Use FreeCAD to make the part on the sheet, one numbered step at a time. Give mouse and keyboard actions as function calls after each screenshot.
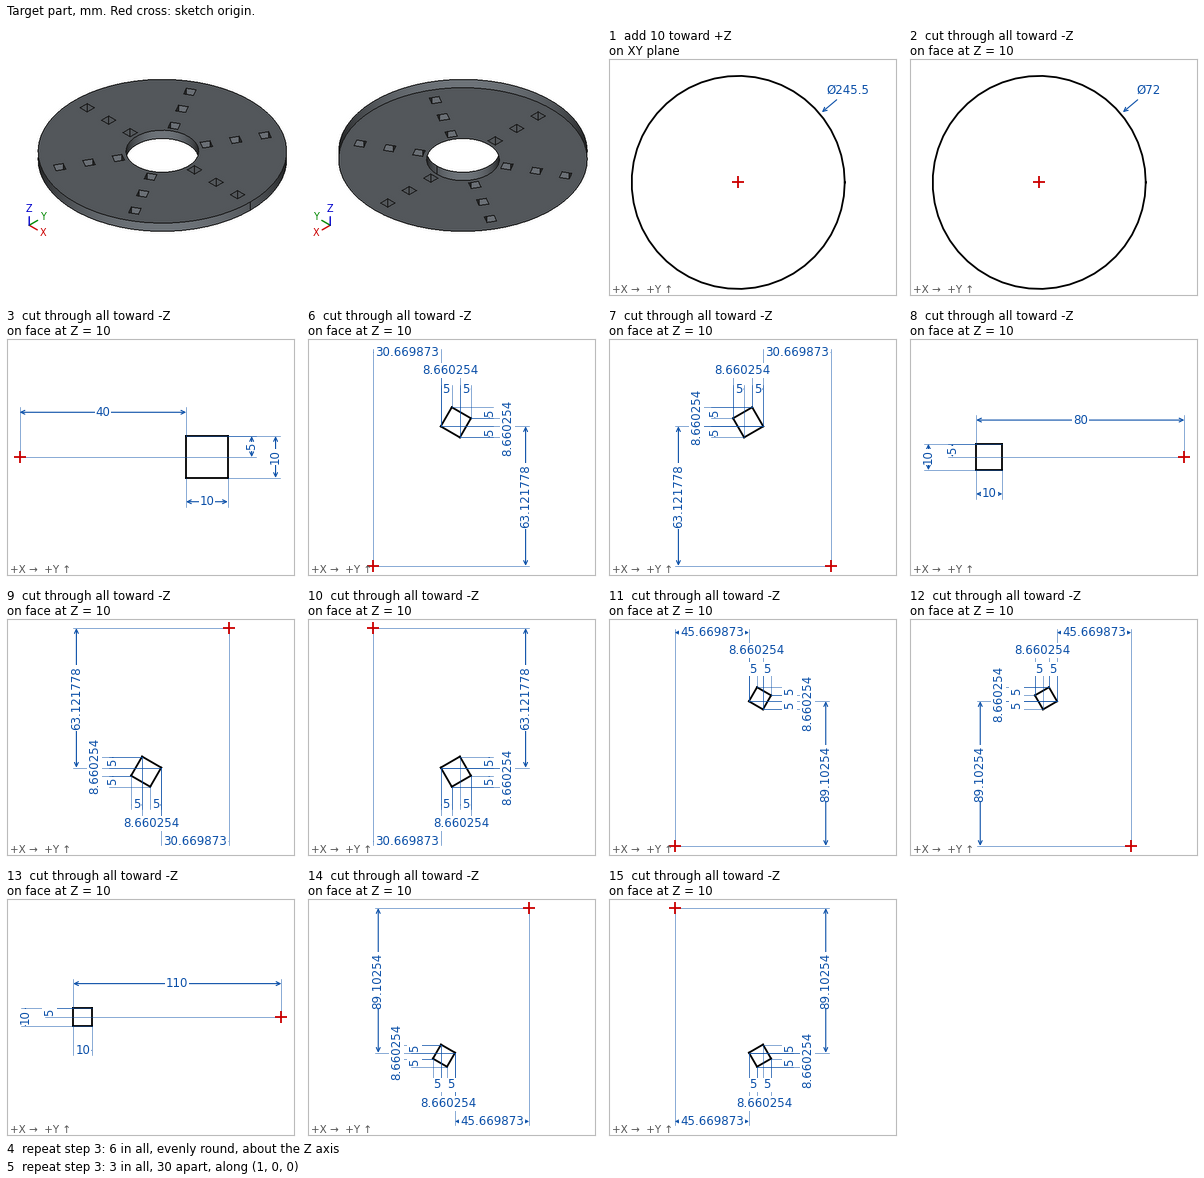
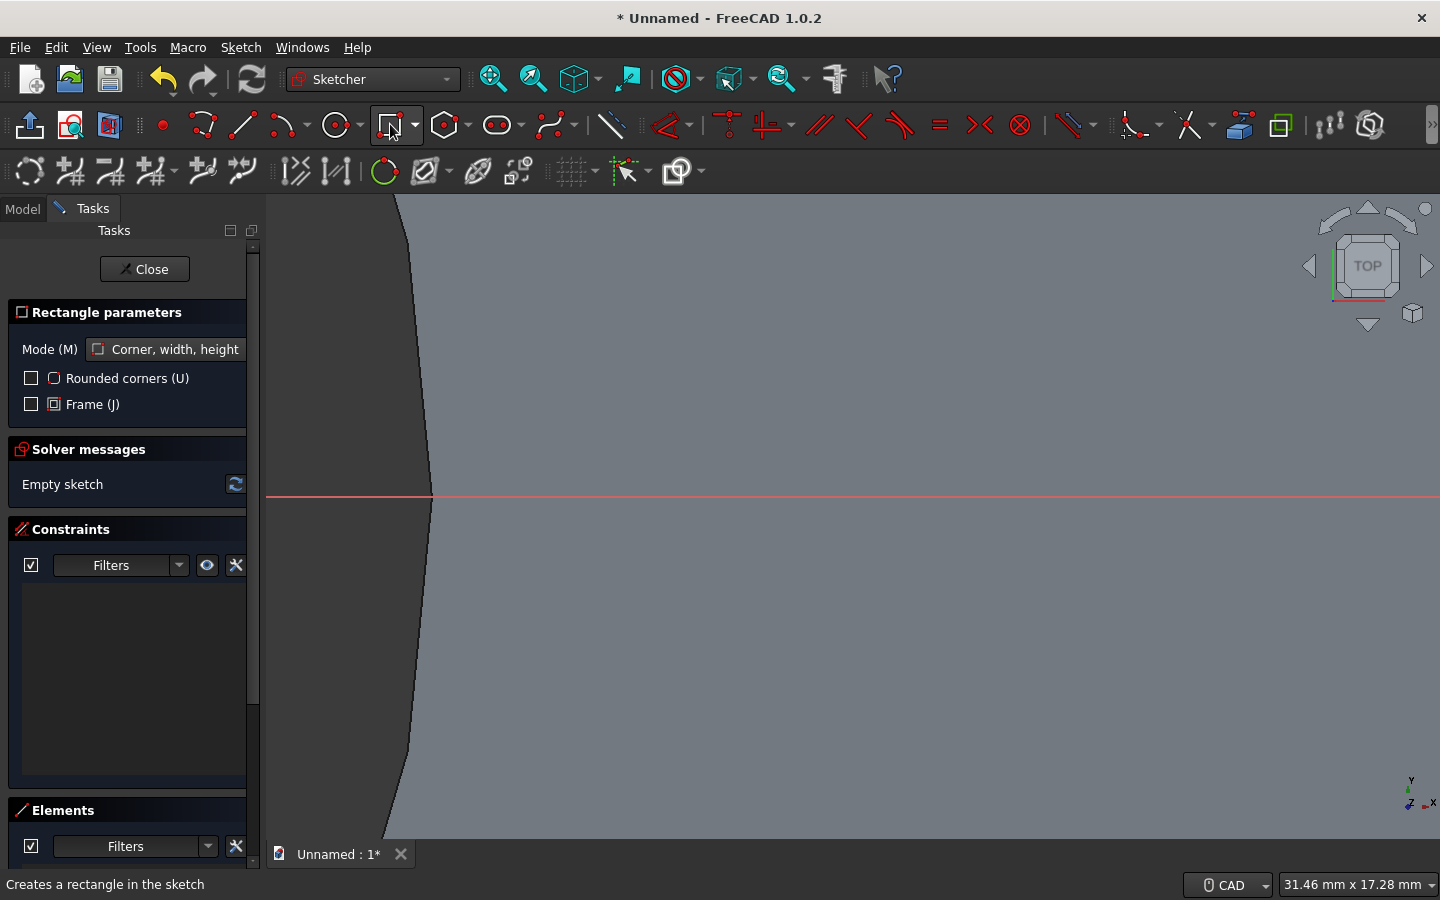
click(581, 311)
move(954, 684)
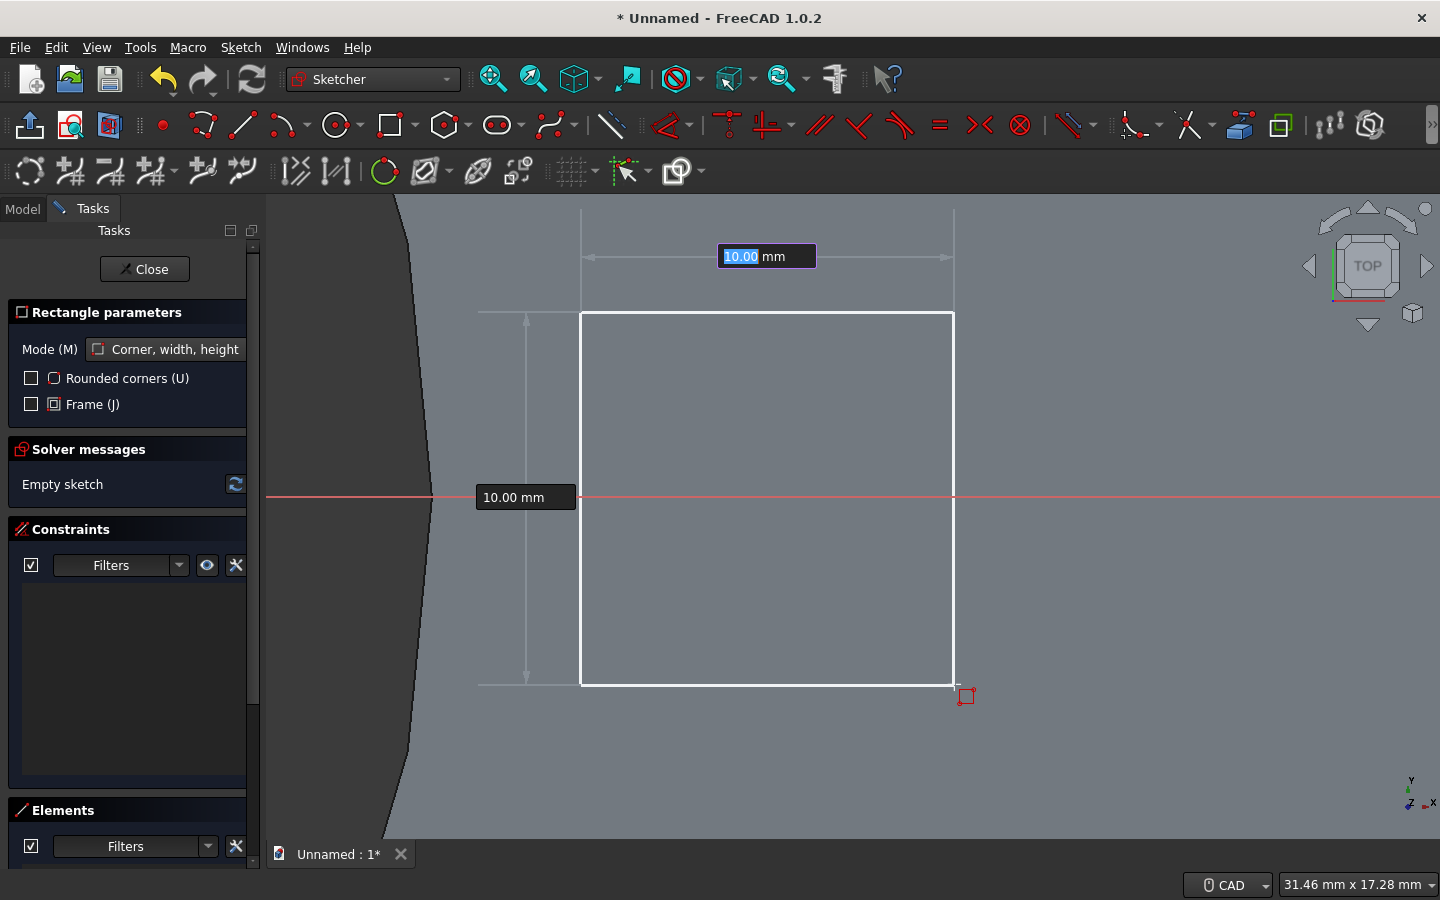
text(10)
key(Tab)
text(10)
key(Return)
key(Escape)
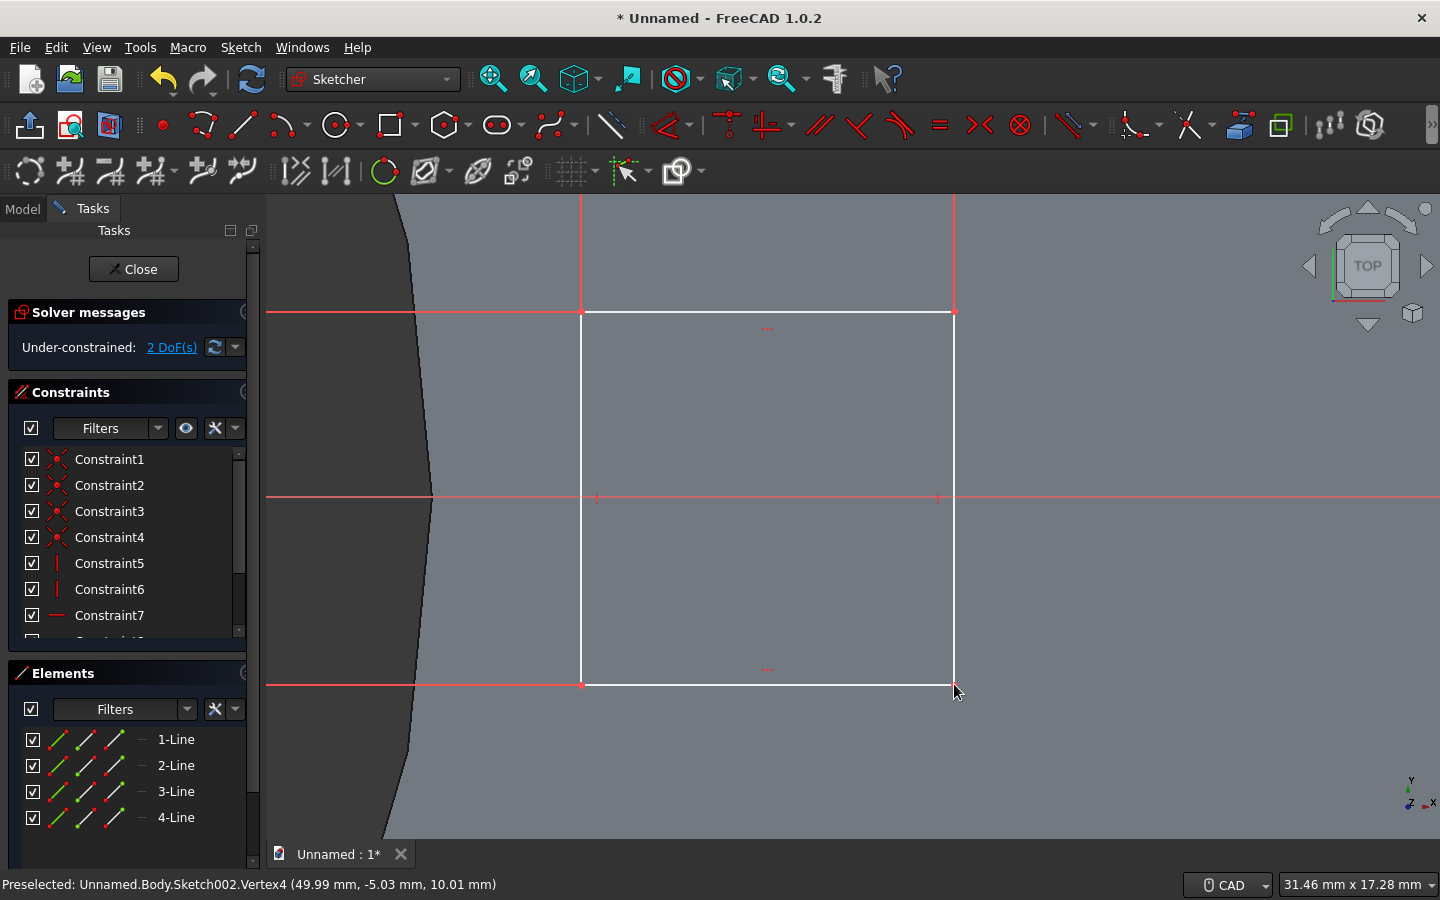
key(d)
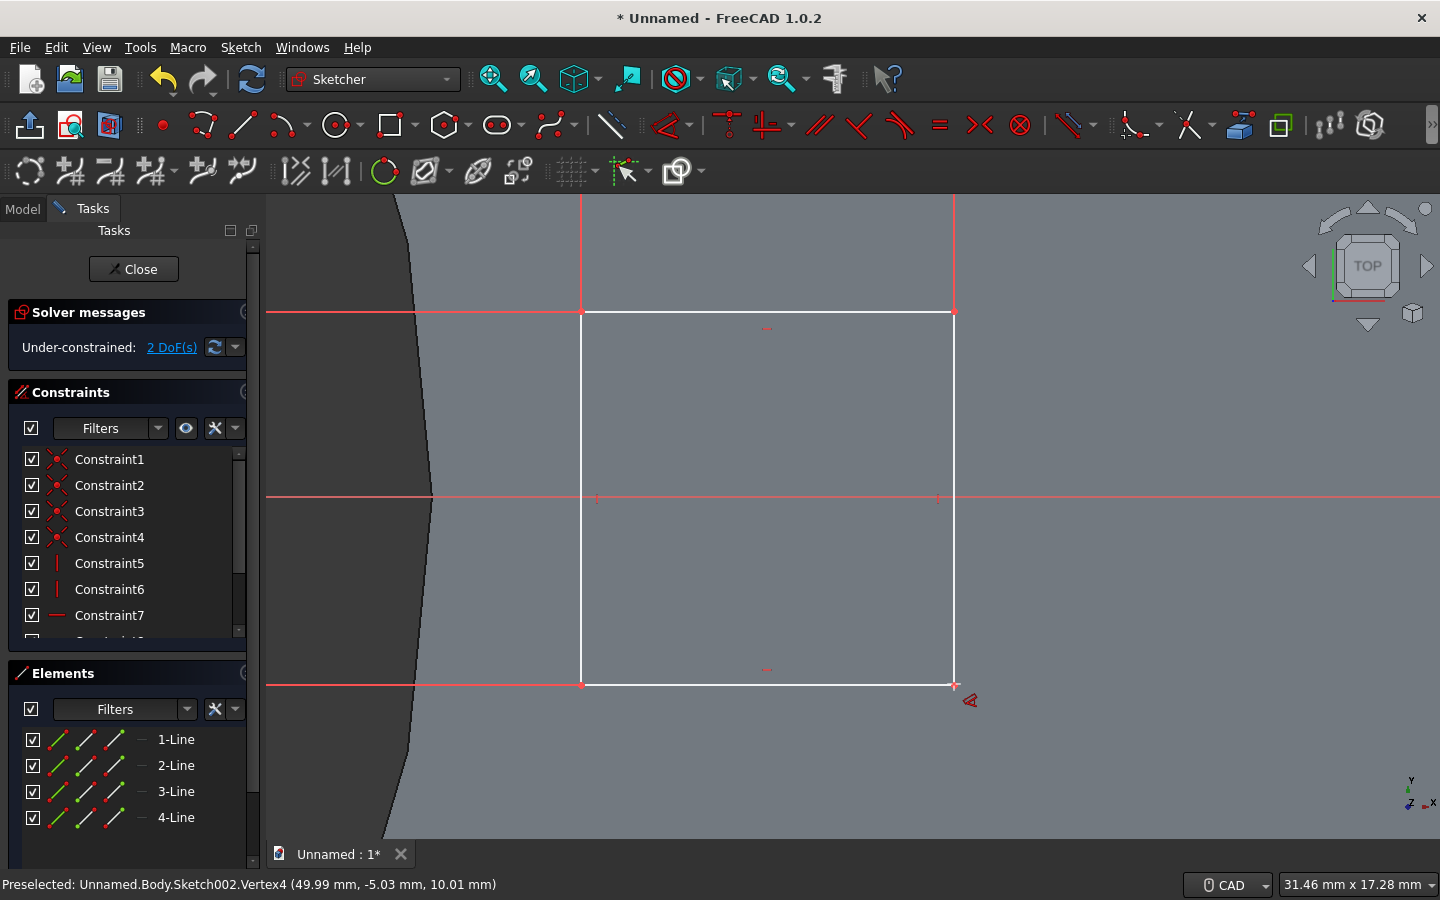
click(581, 312)
click(615, 405)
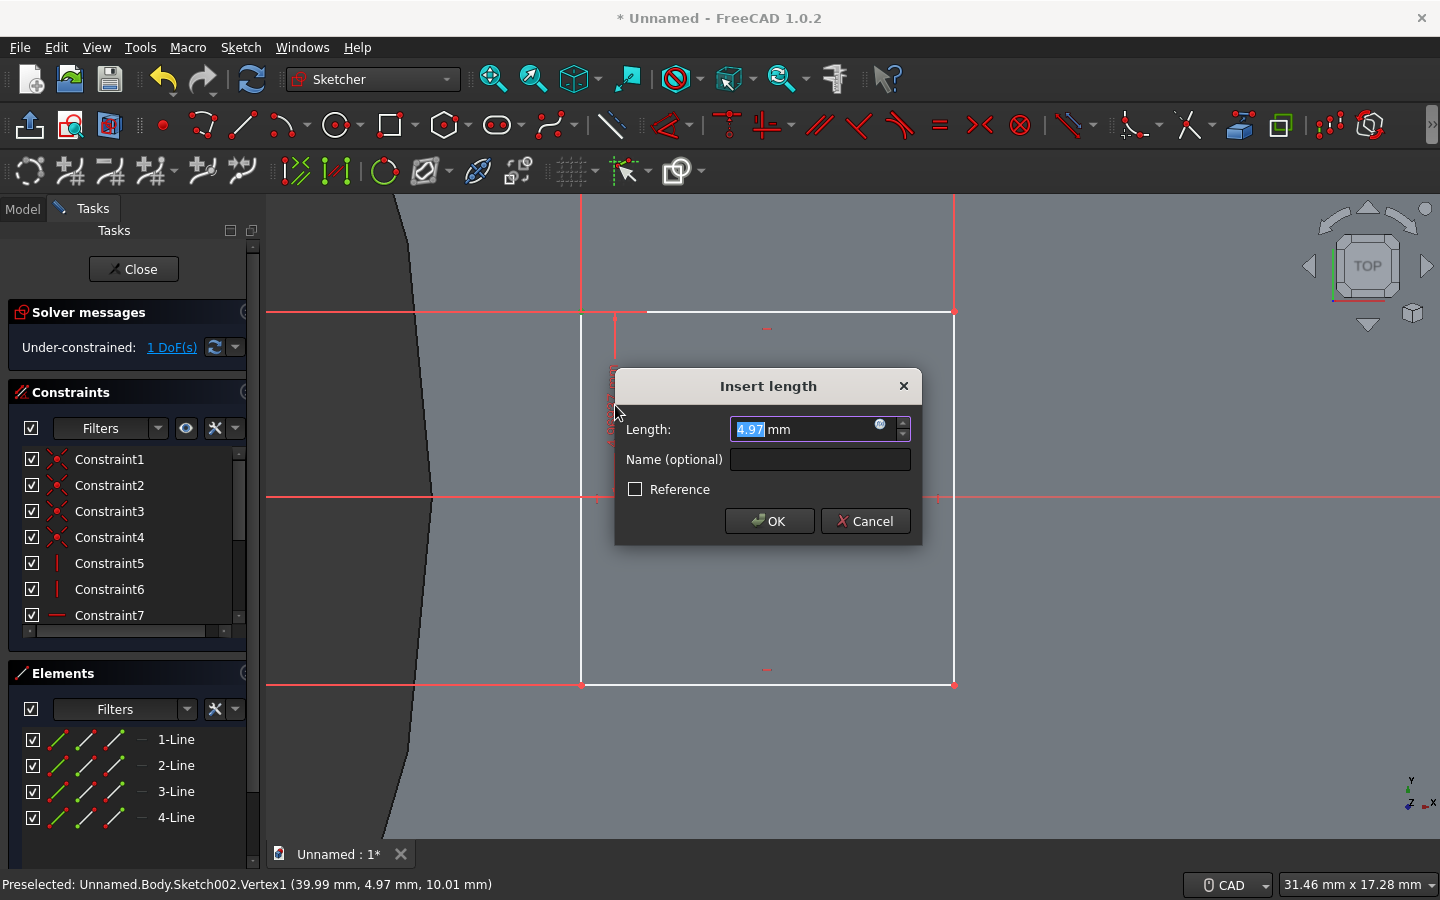
text(5)
key(Return)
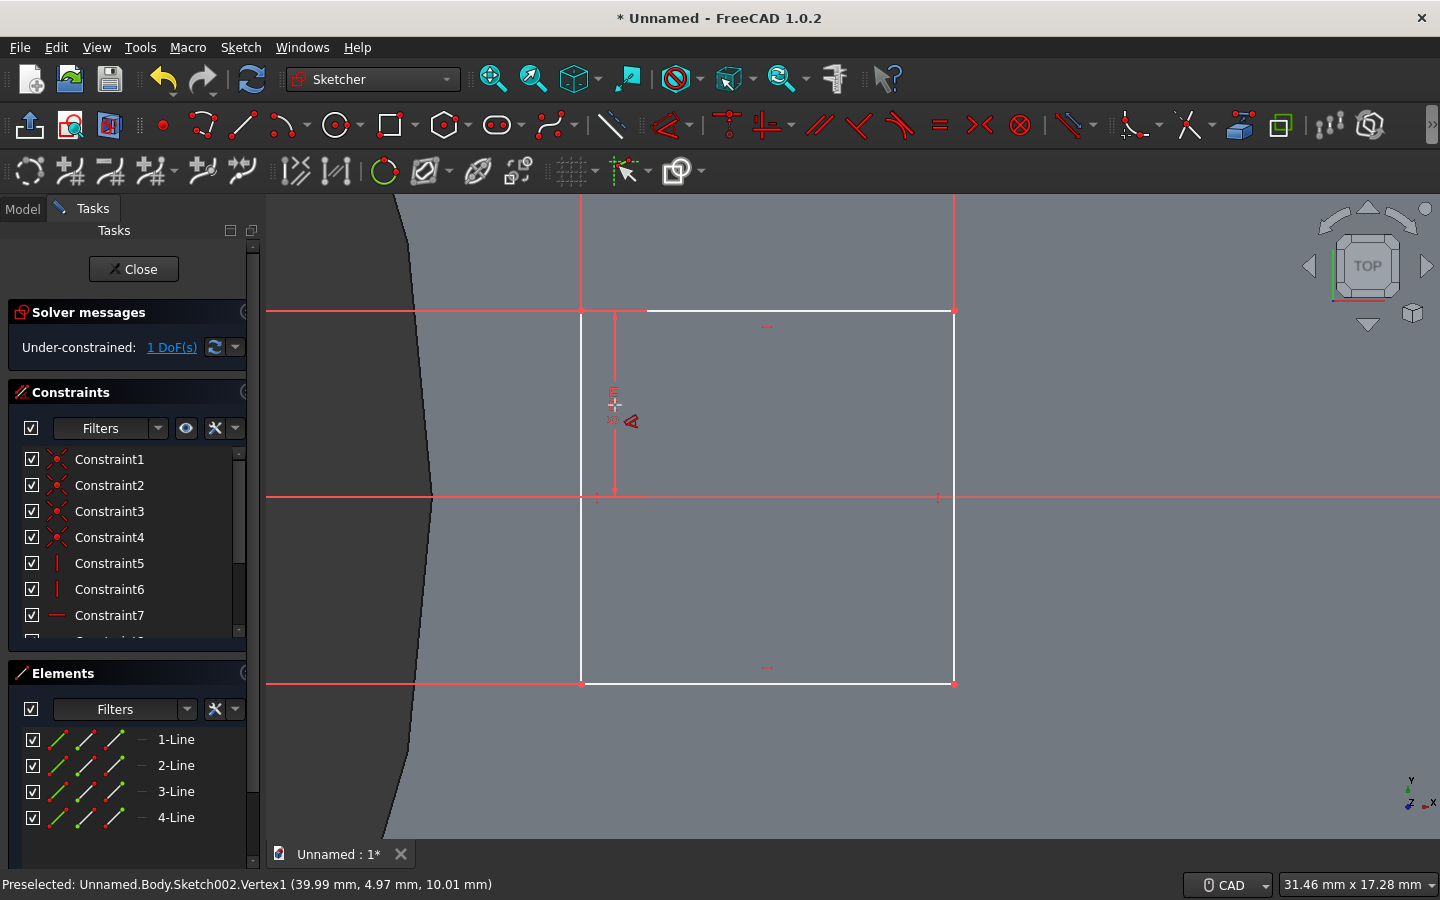
click(581, 311)
click(437, 277)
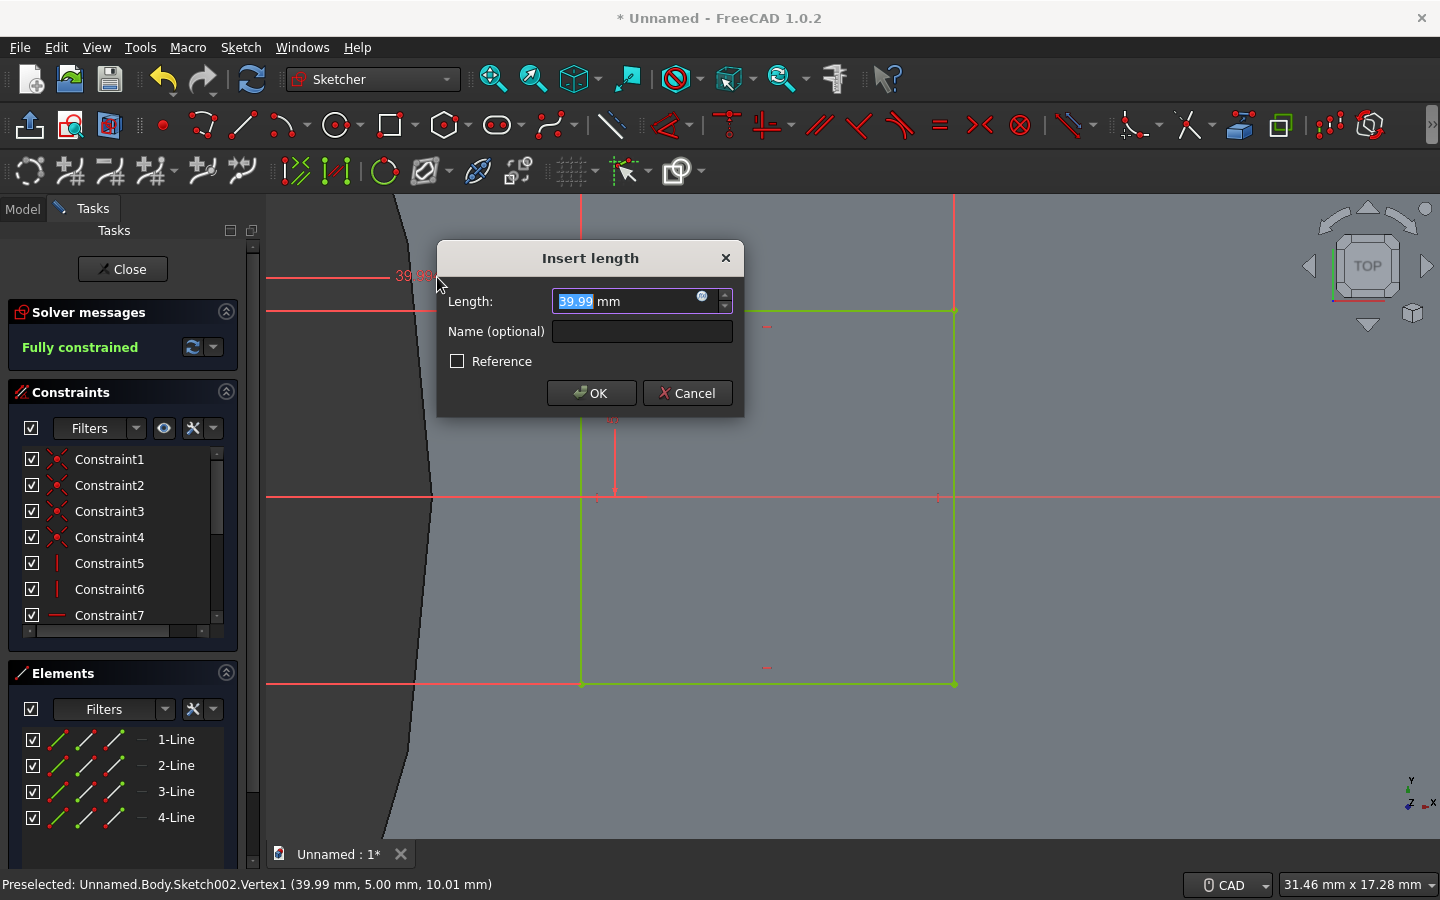
text(40)
key(Return)
key(Escape)